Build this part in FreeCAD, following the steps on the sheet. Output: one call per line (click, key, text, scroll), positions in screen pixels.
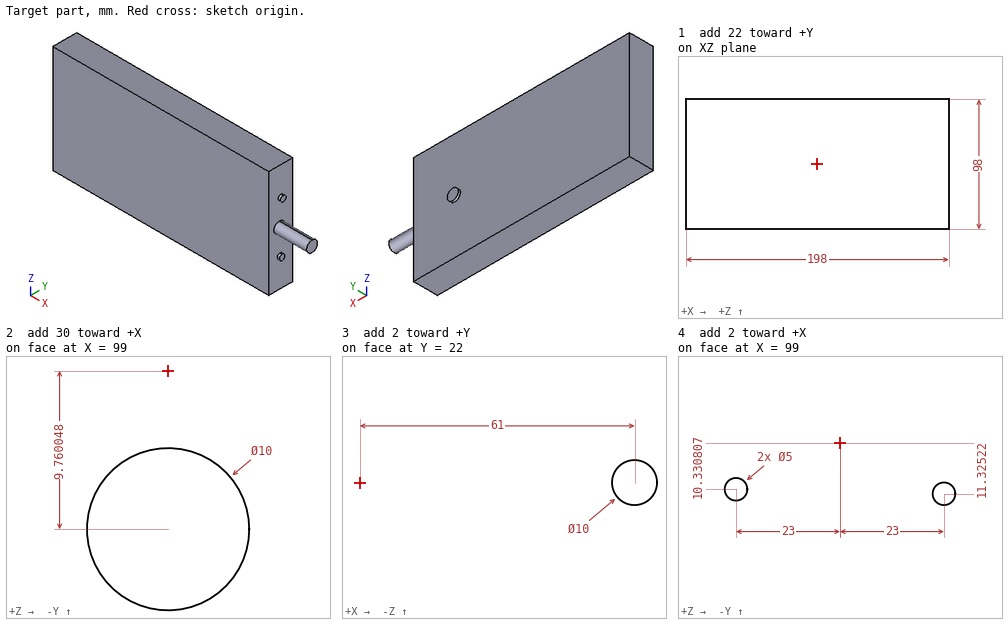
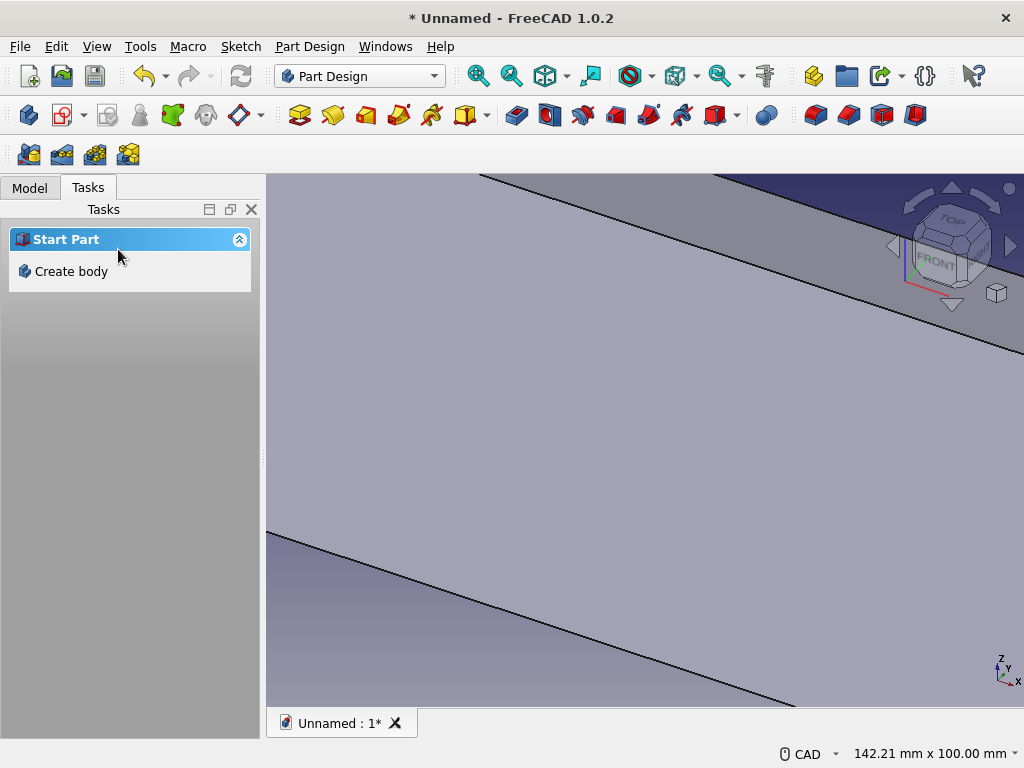
click(479, 76)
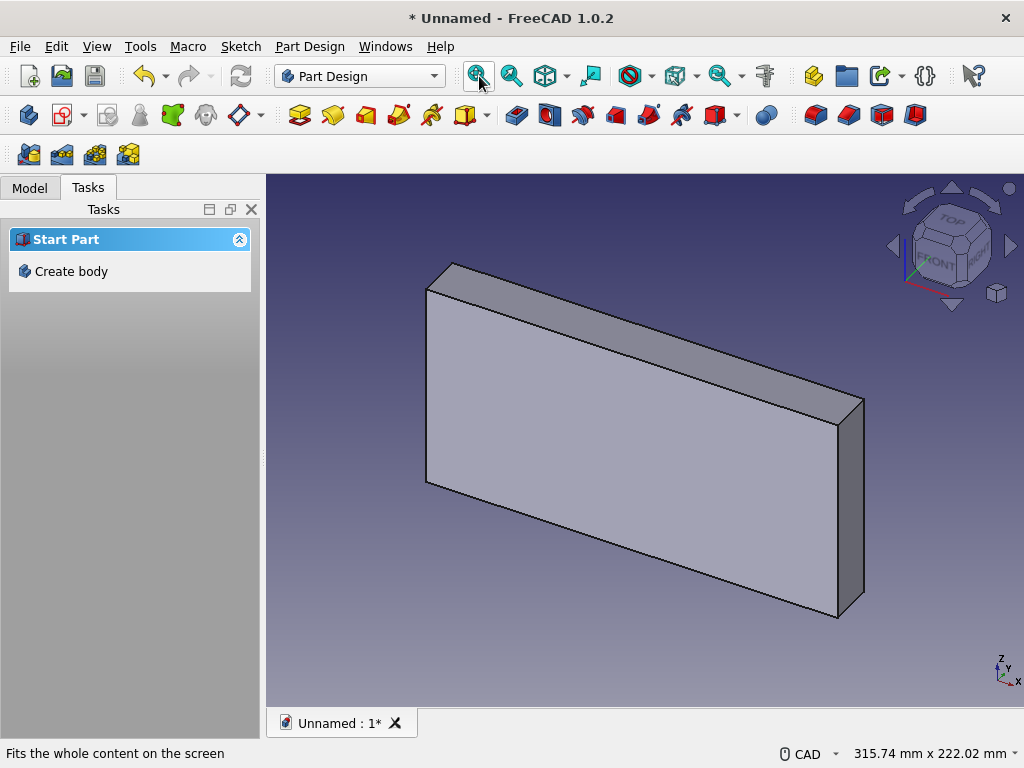
click(851, 453)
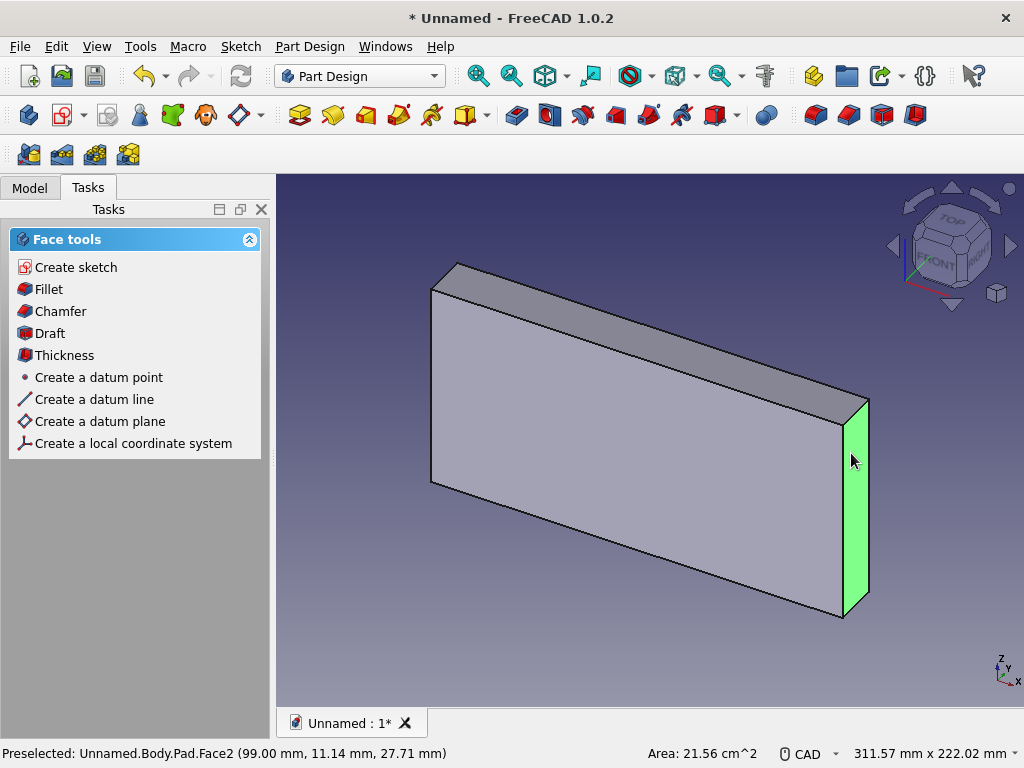
click(62, 116)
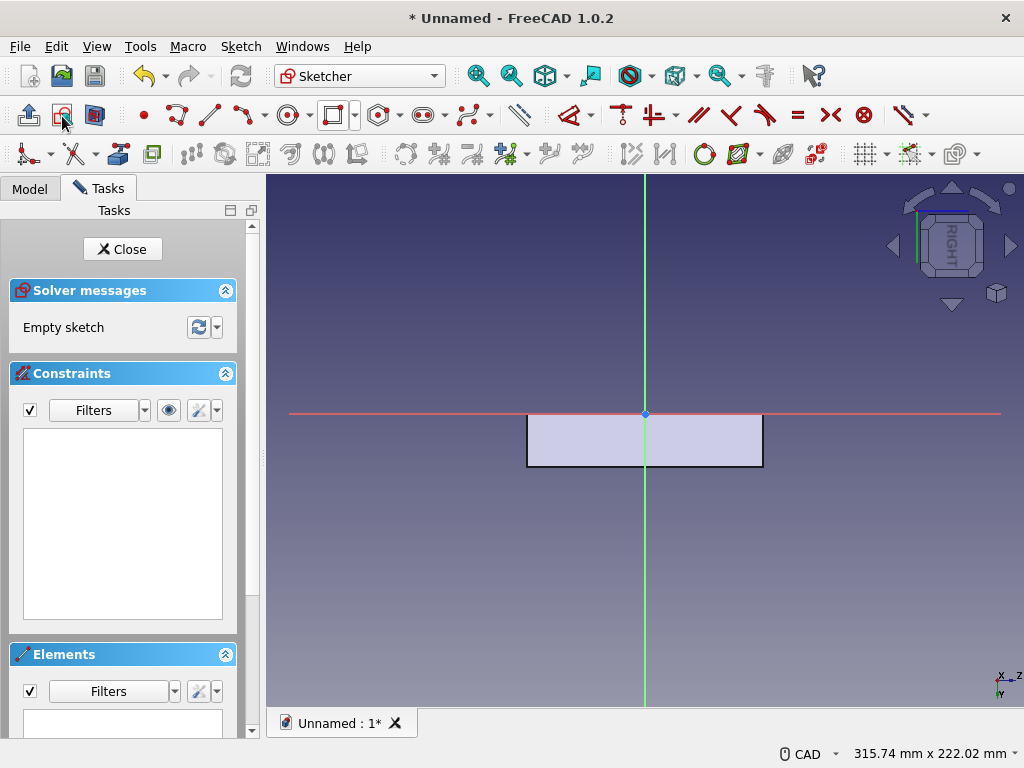
scroll(654, 431, up, 11)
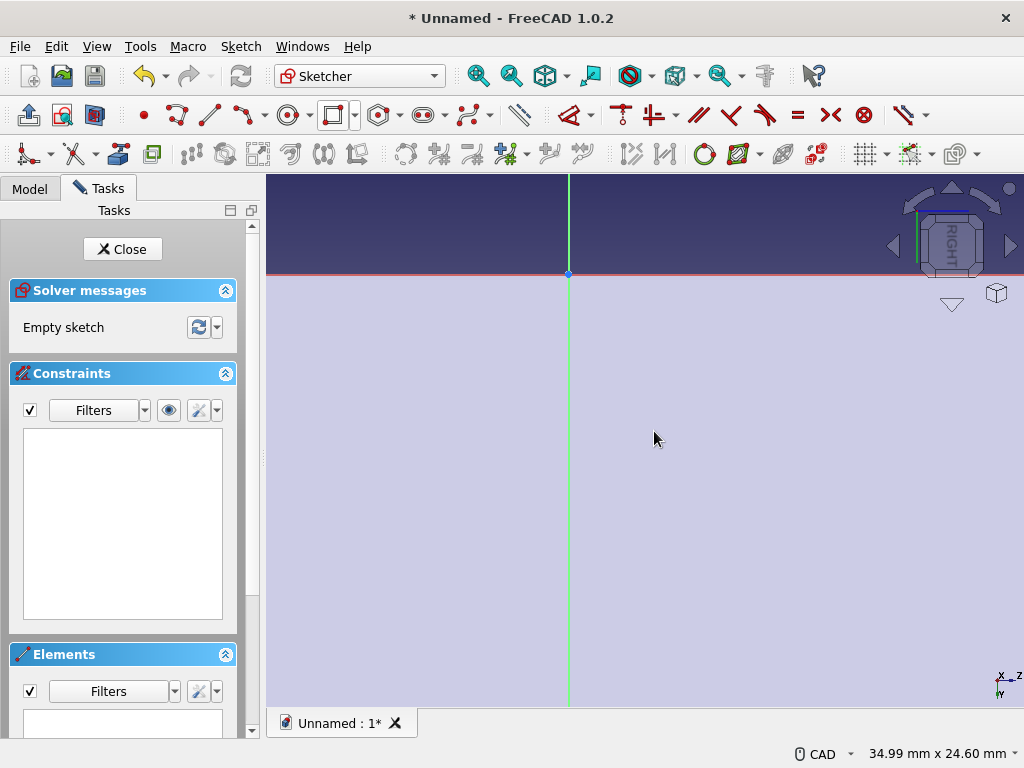
key(g)
key(c)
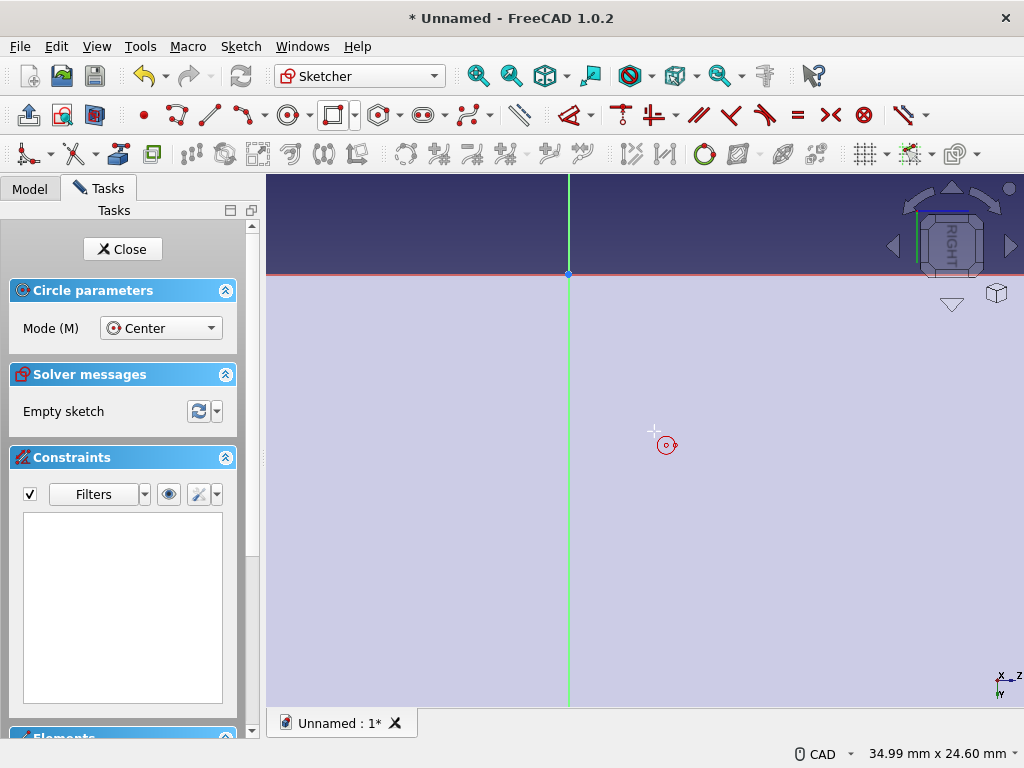
click(569, 486)
move(645, 409)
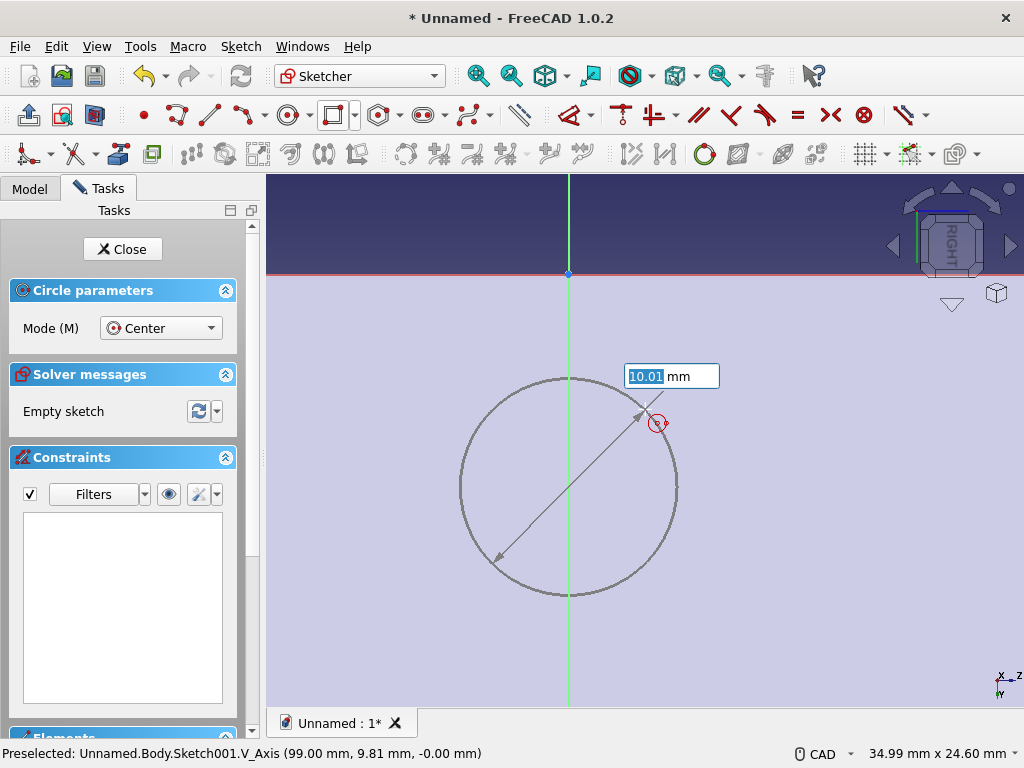
text(10)
key(Return)
key(Escape)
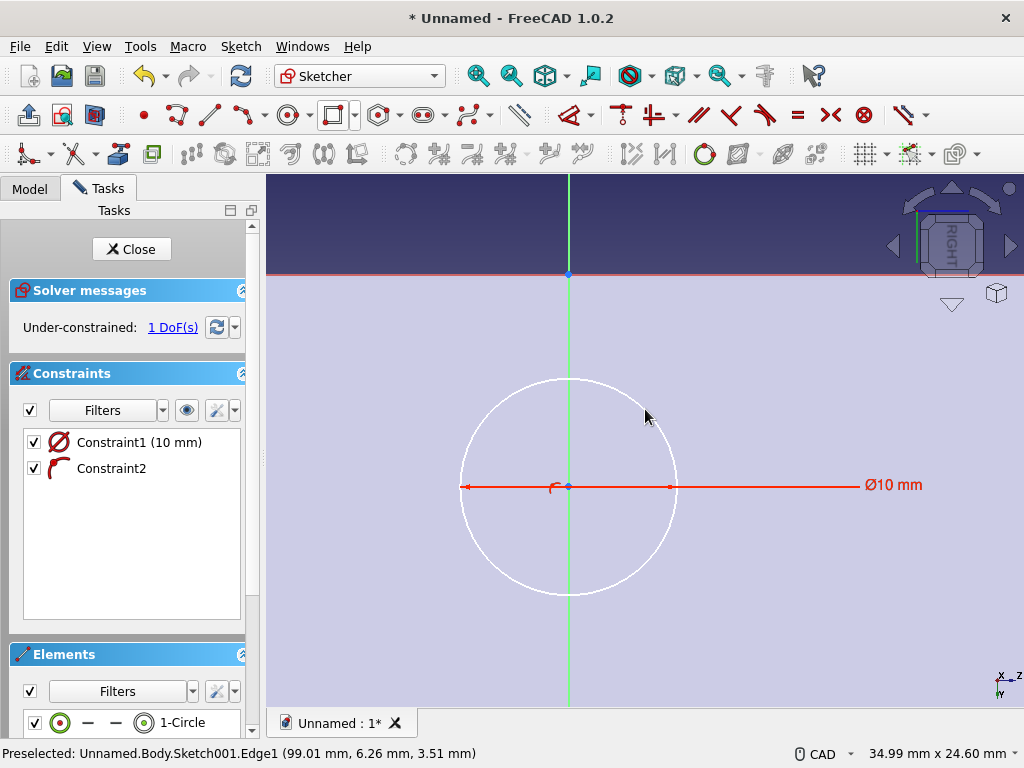
click(568, 116)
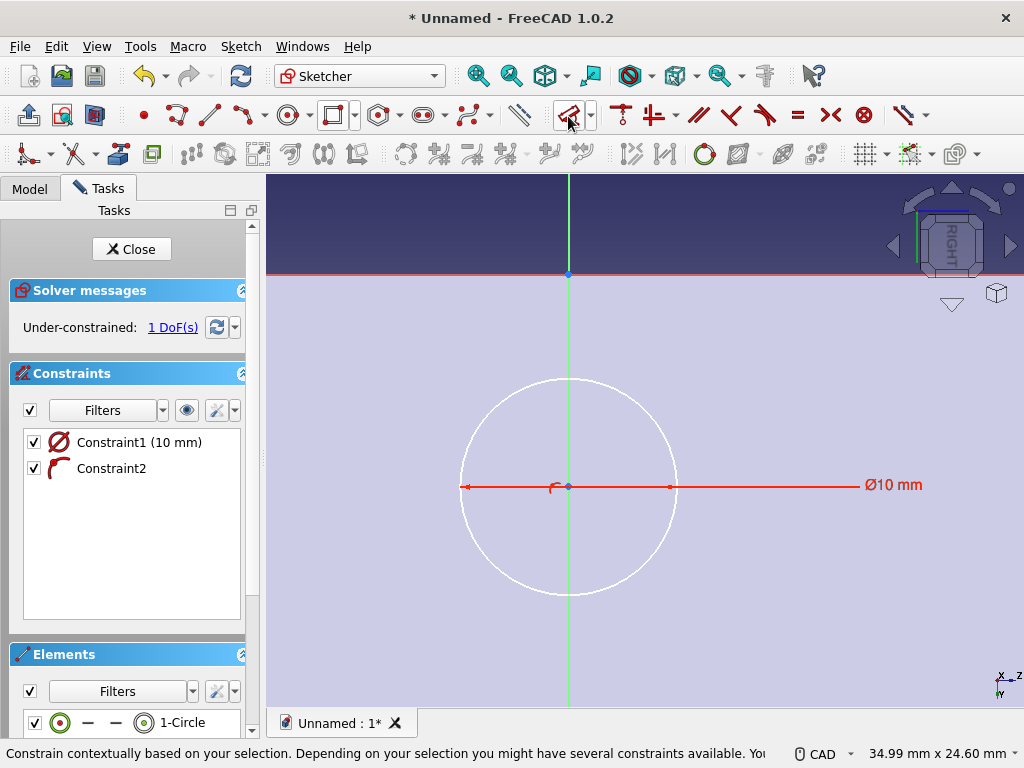
click(569, 487)
click(603, 332)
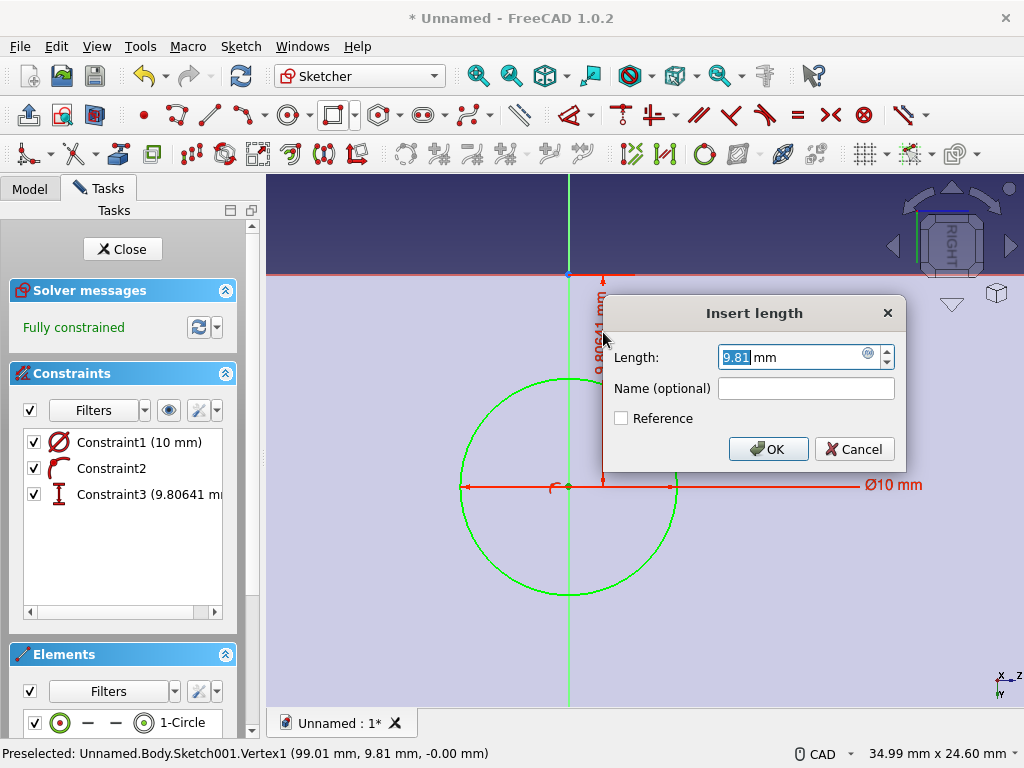
text(9.760048)
key(Return)
key(Escape)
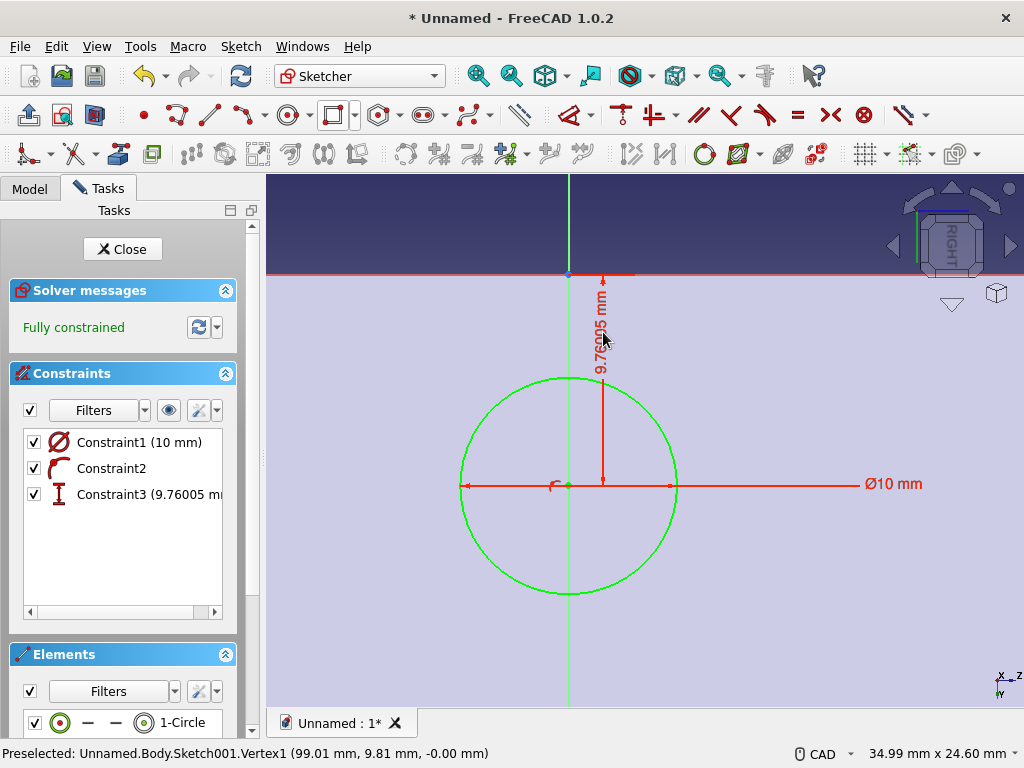
click(123, 249)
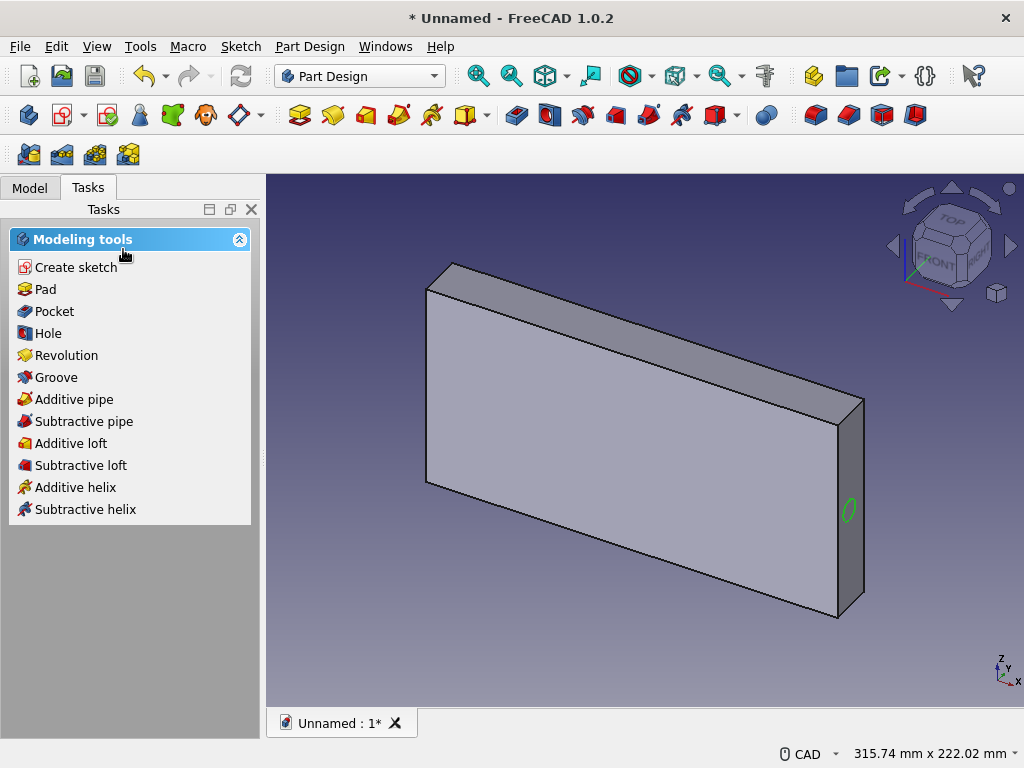
click(300, 116)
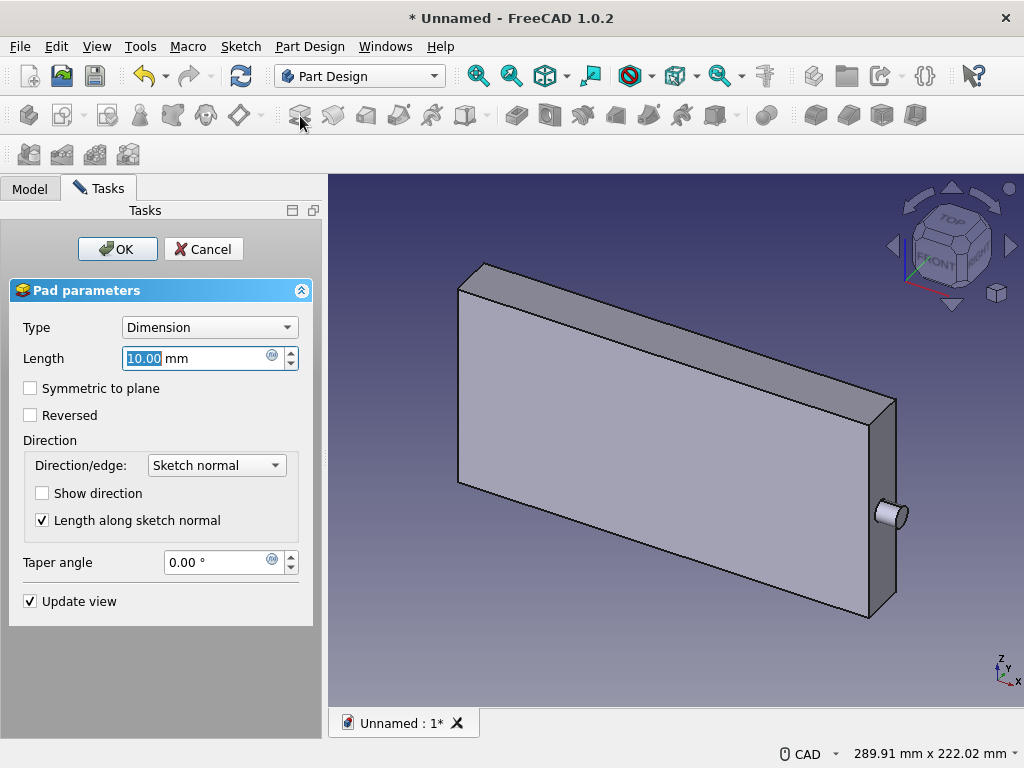
text(30)
key(Tab)